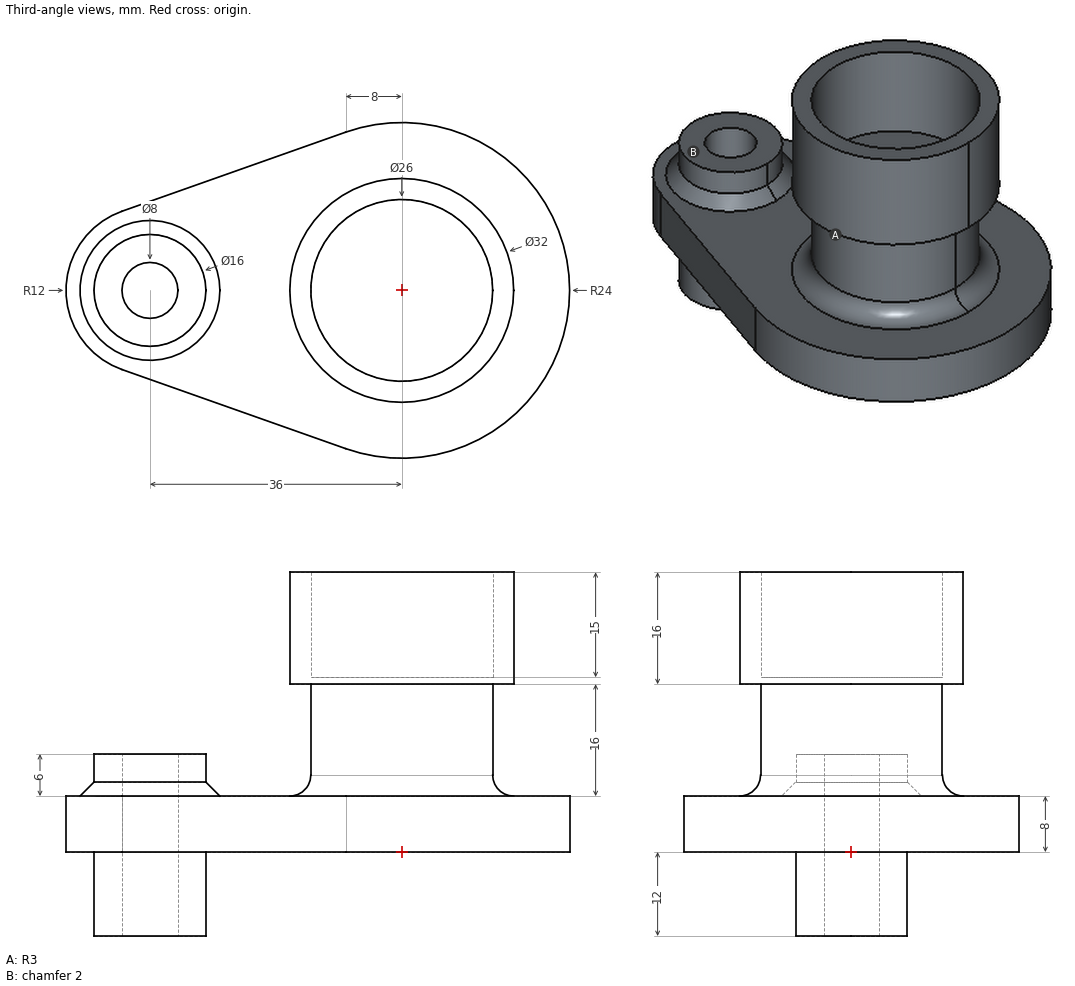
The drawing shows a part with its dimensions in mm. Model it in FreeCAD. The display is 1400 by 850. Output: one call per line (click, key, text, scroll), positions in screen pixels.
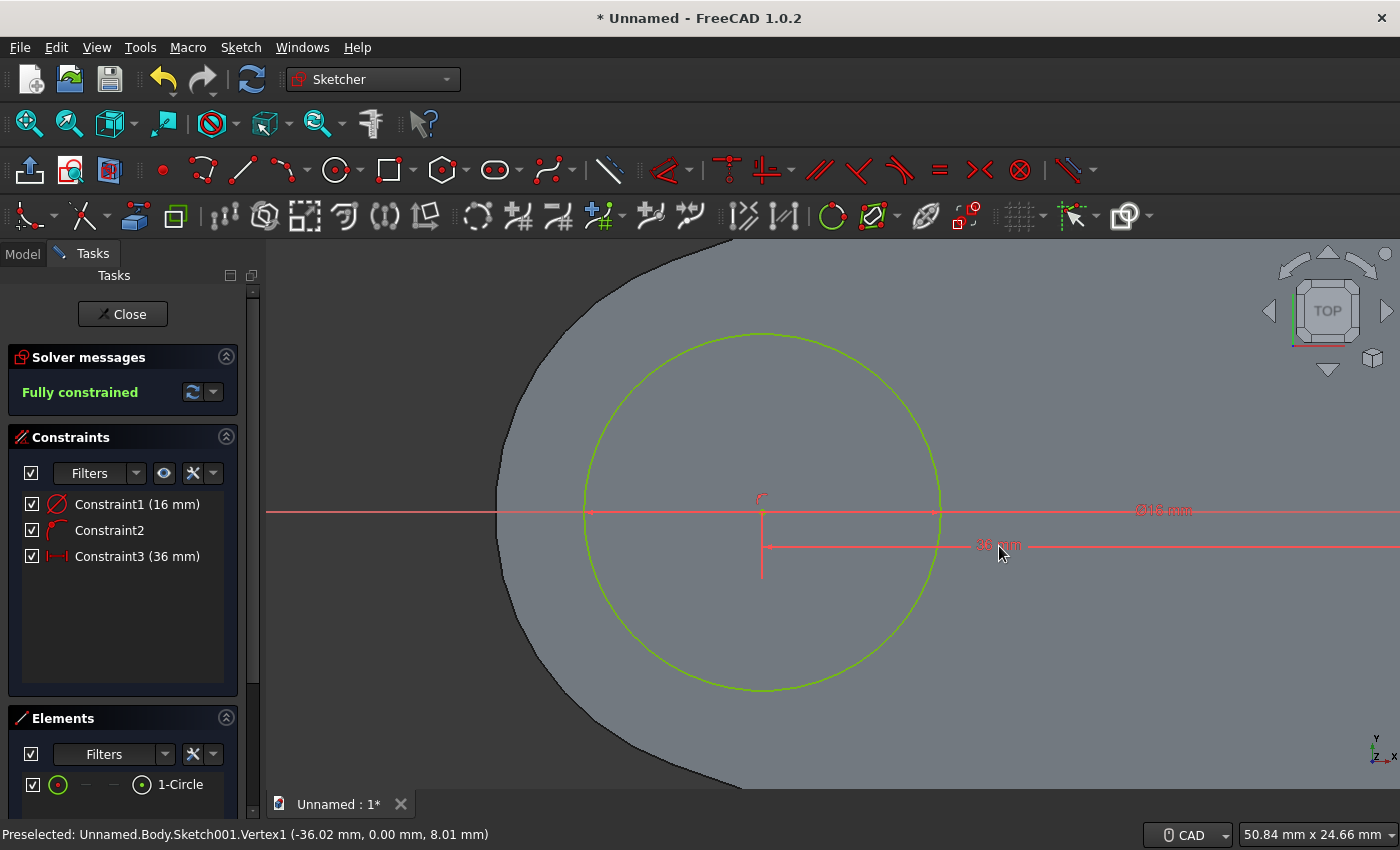
click(123, 314)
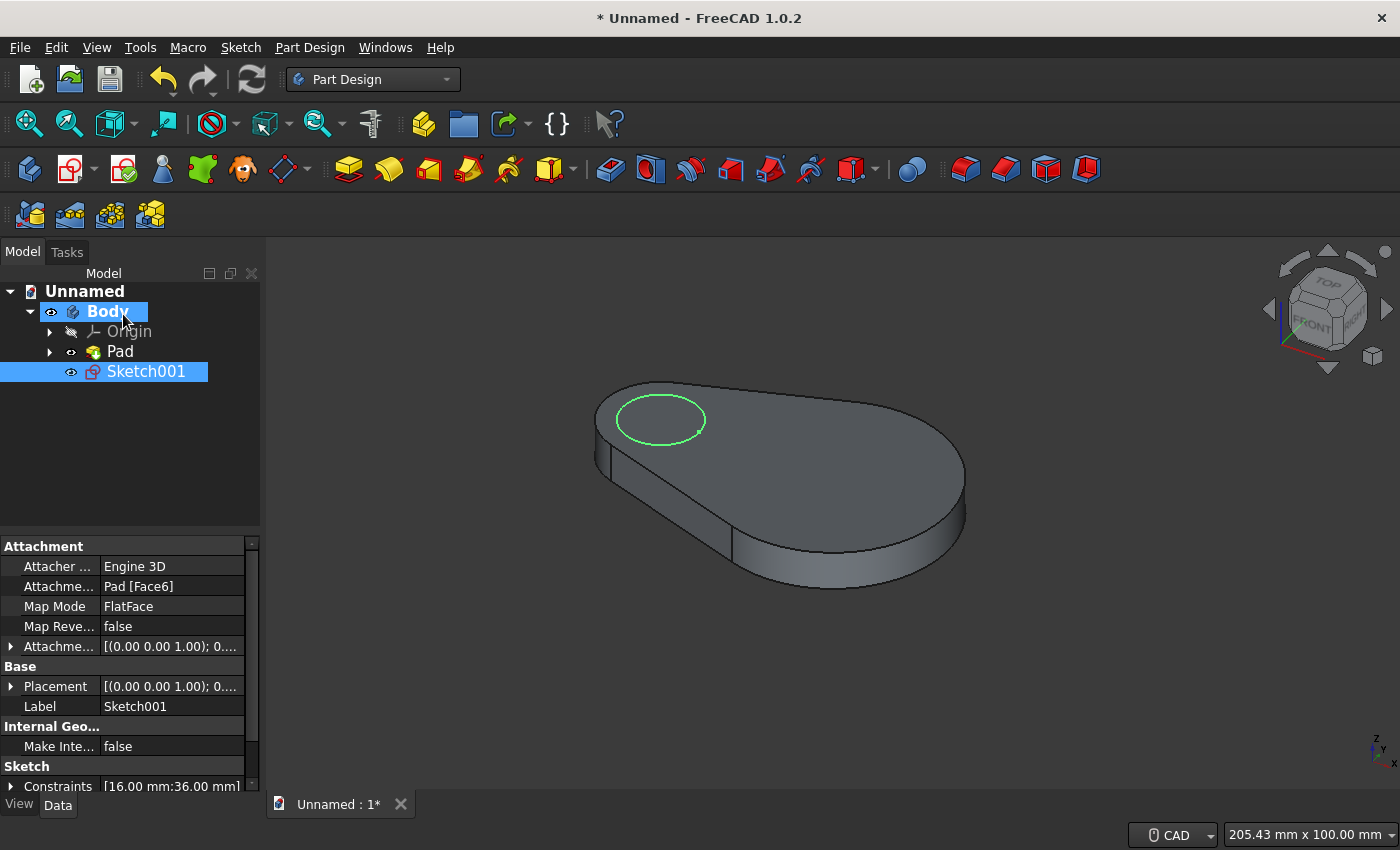
click(350, 170)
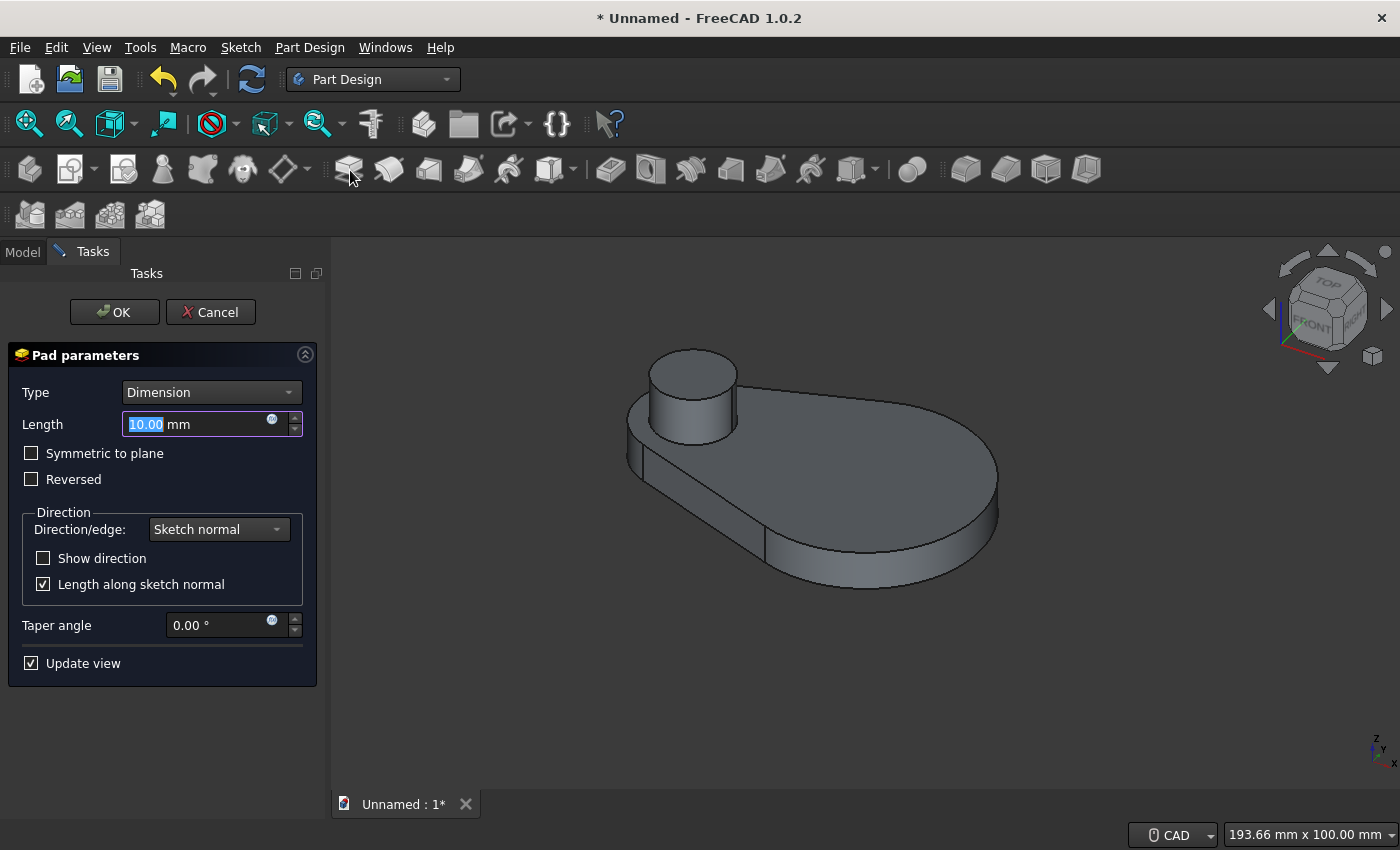
text(6)
key(Tab)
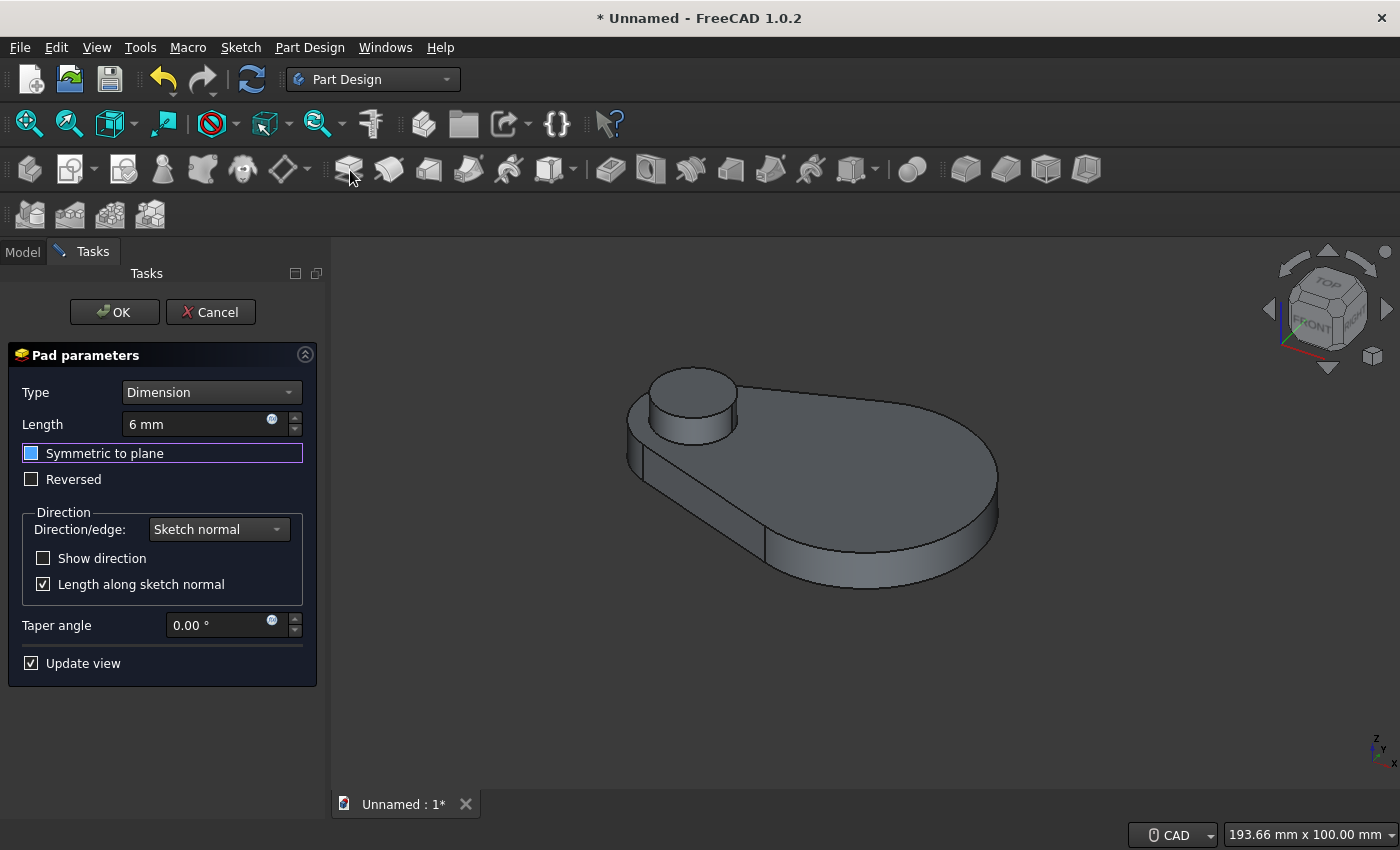
click(115, 312)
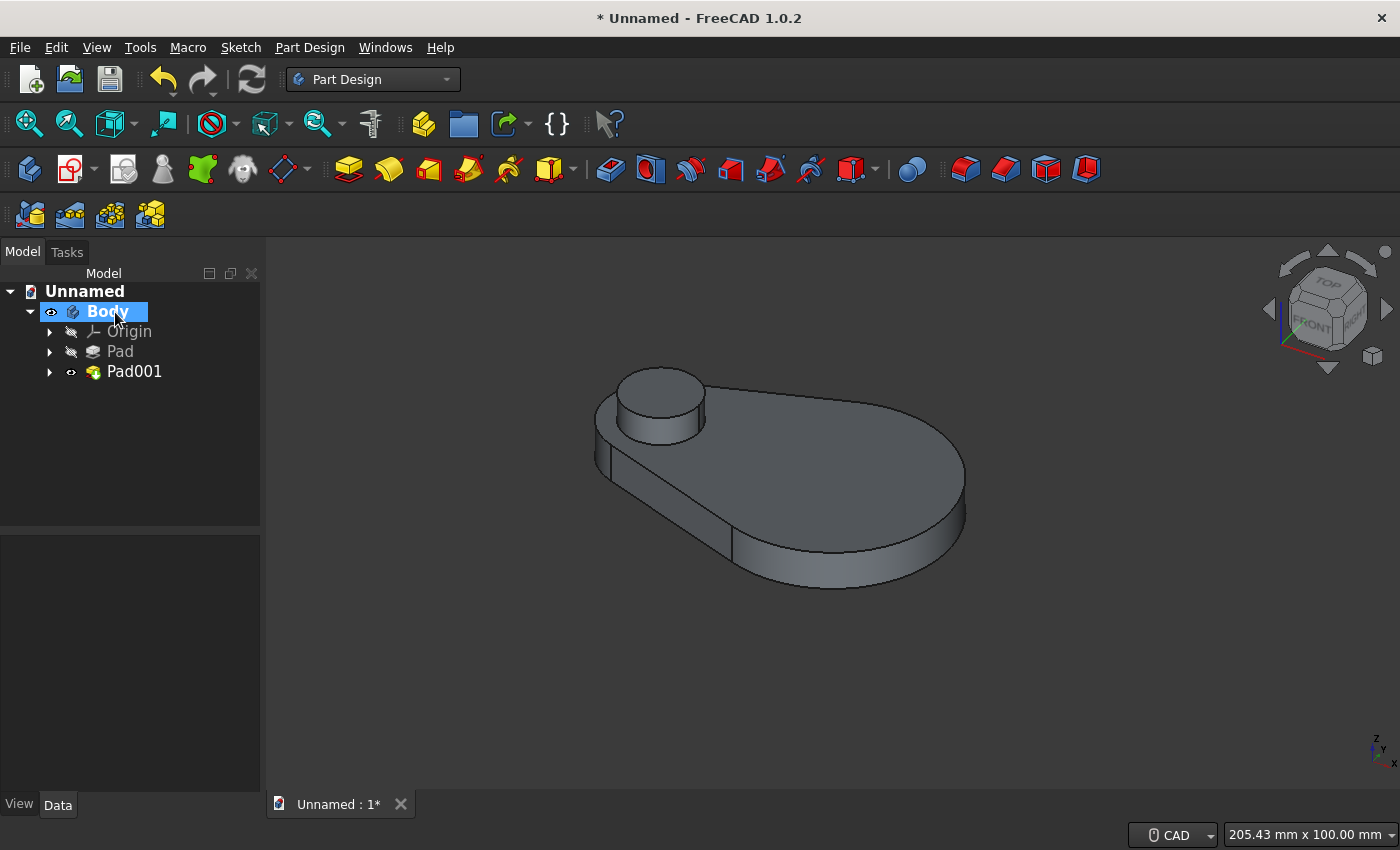
click(50, 332)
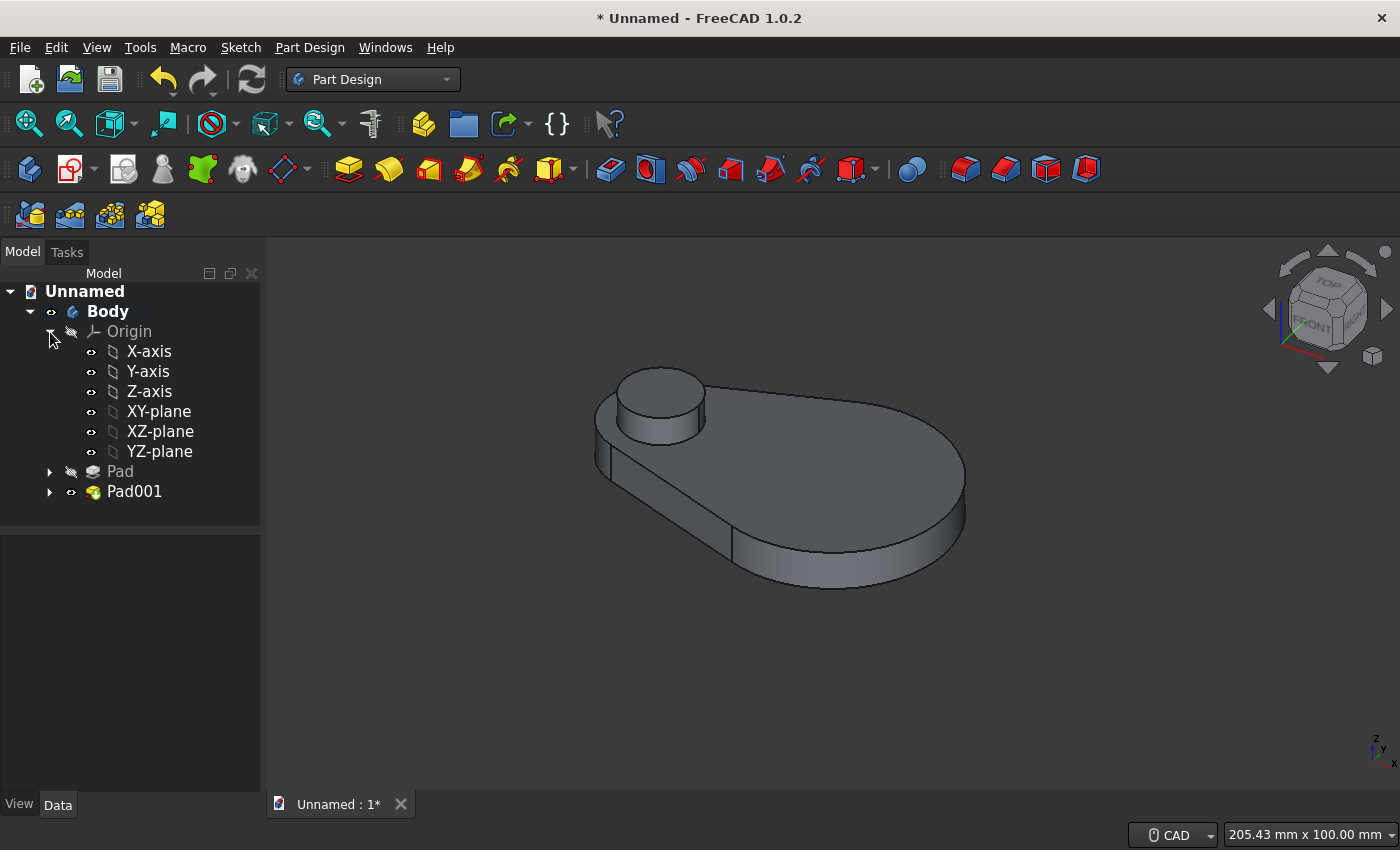
click(136, 412)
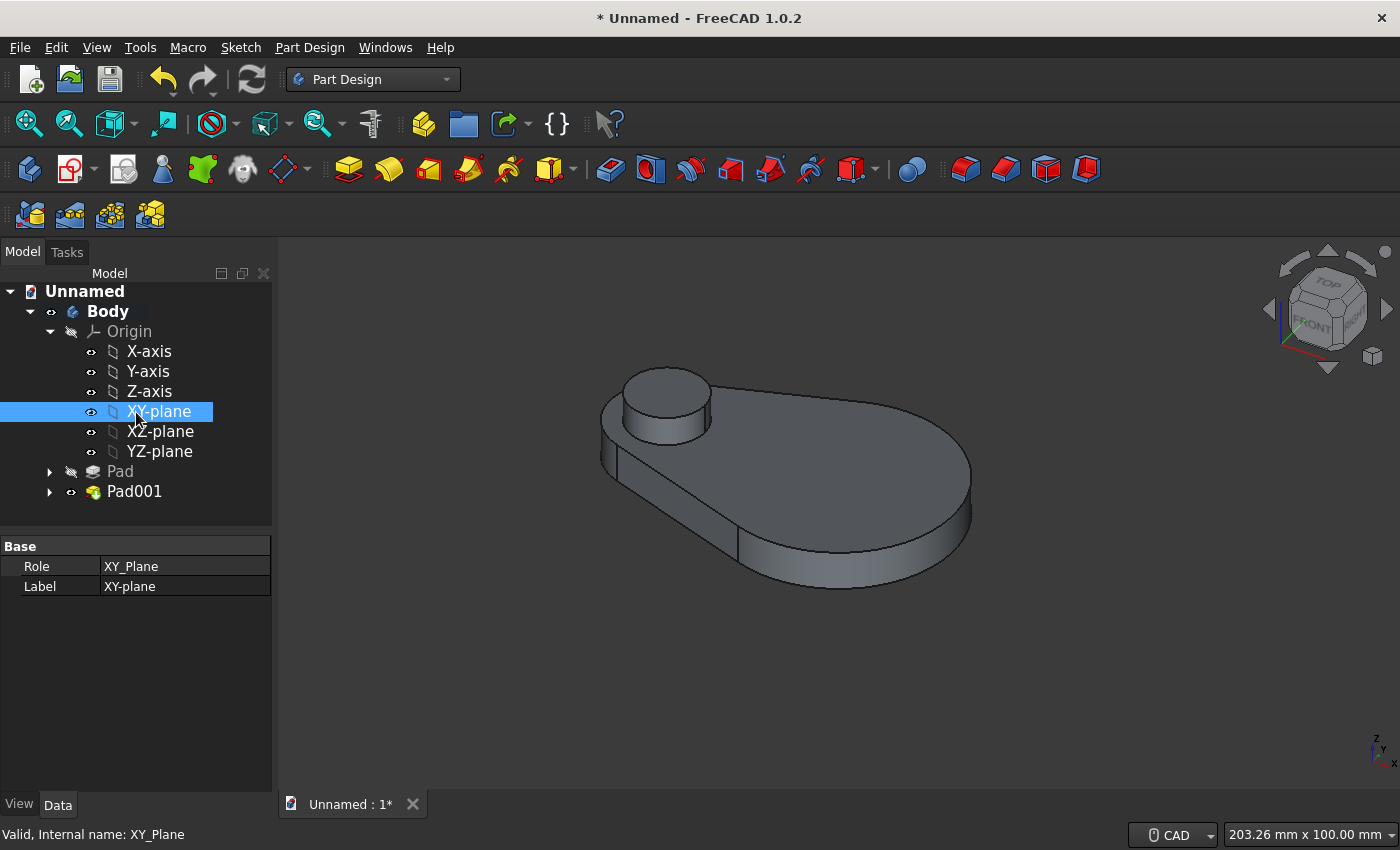
click(284, 170)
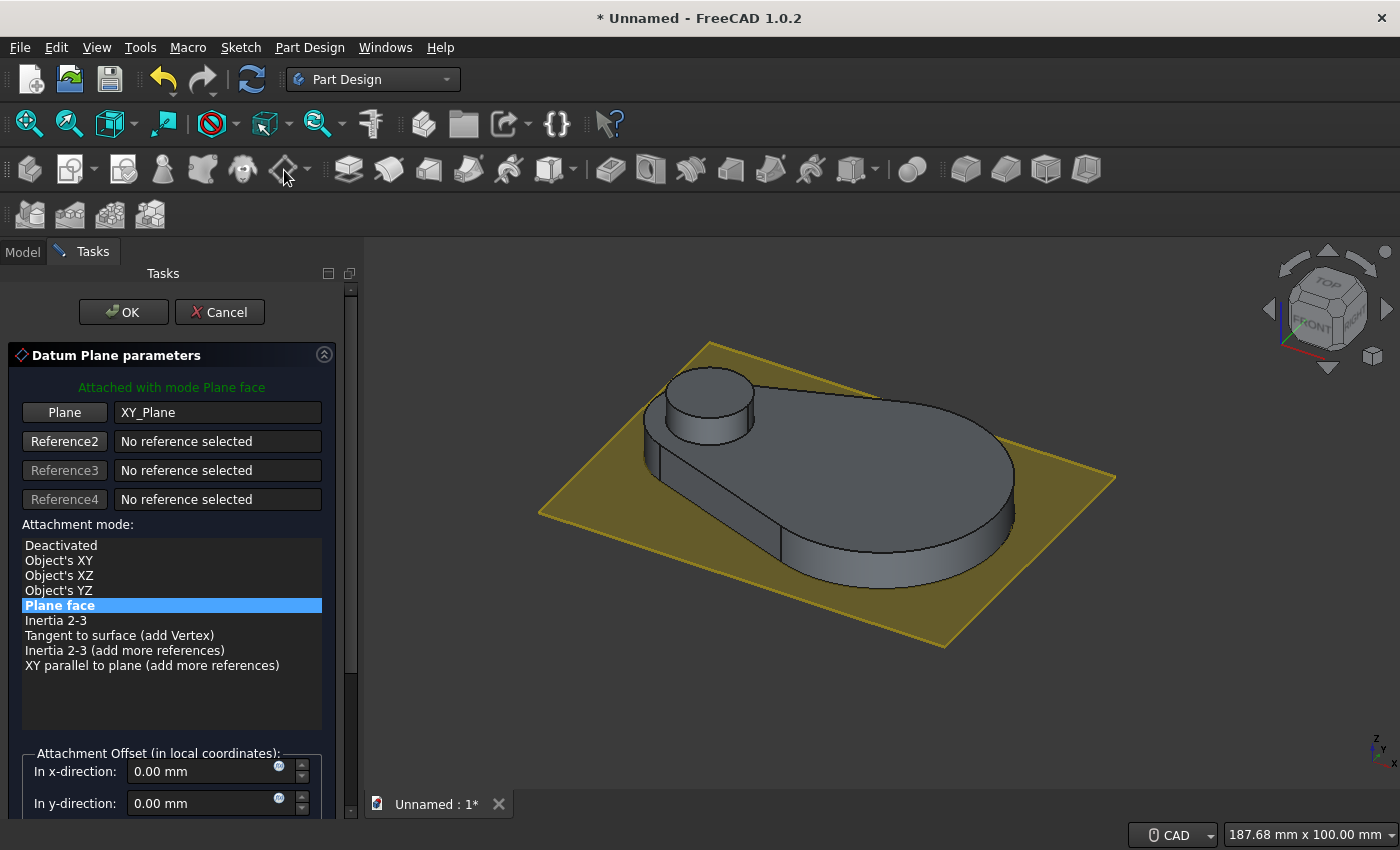
scroll(351, 550, down, 2)